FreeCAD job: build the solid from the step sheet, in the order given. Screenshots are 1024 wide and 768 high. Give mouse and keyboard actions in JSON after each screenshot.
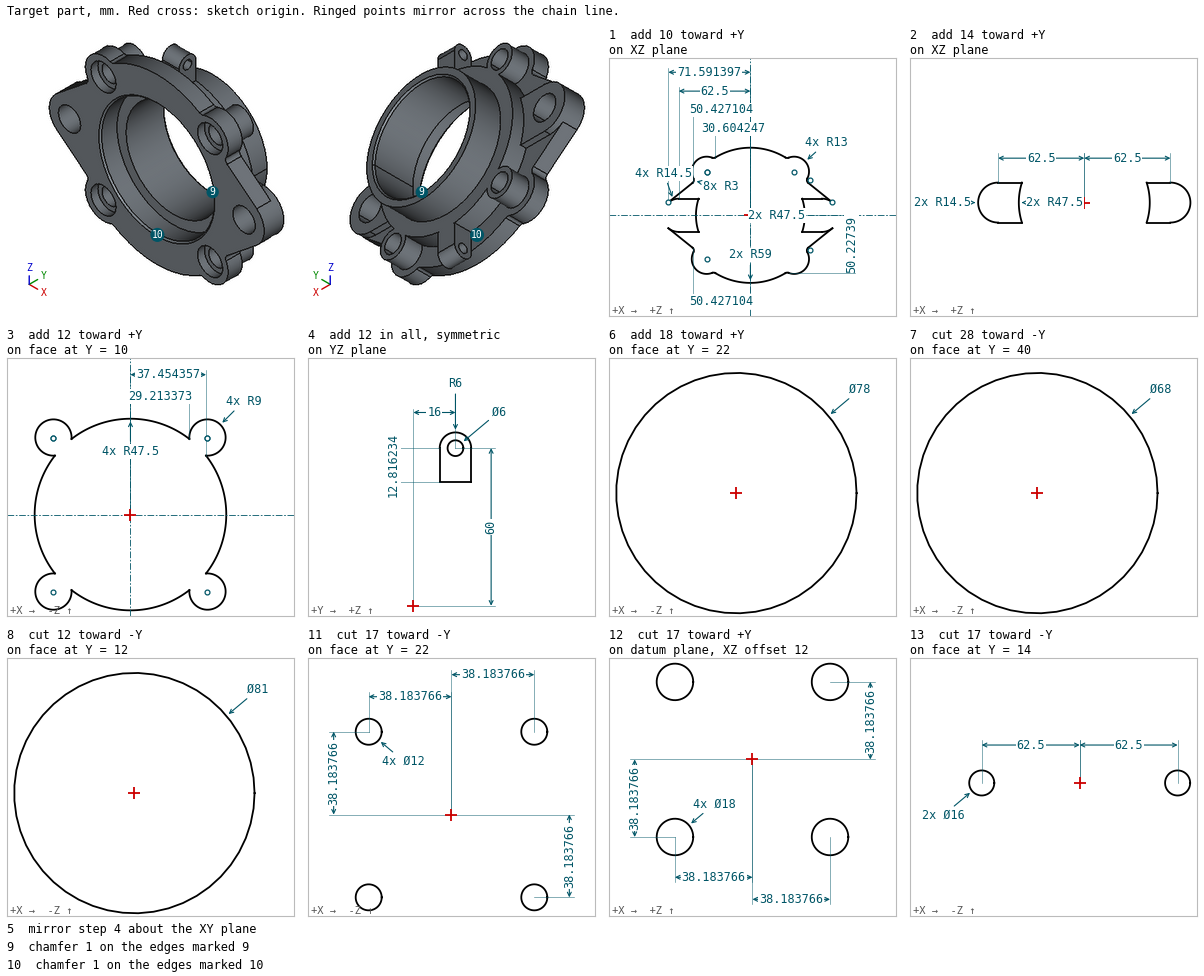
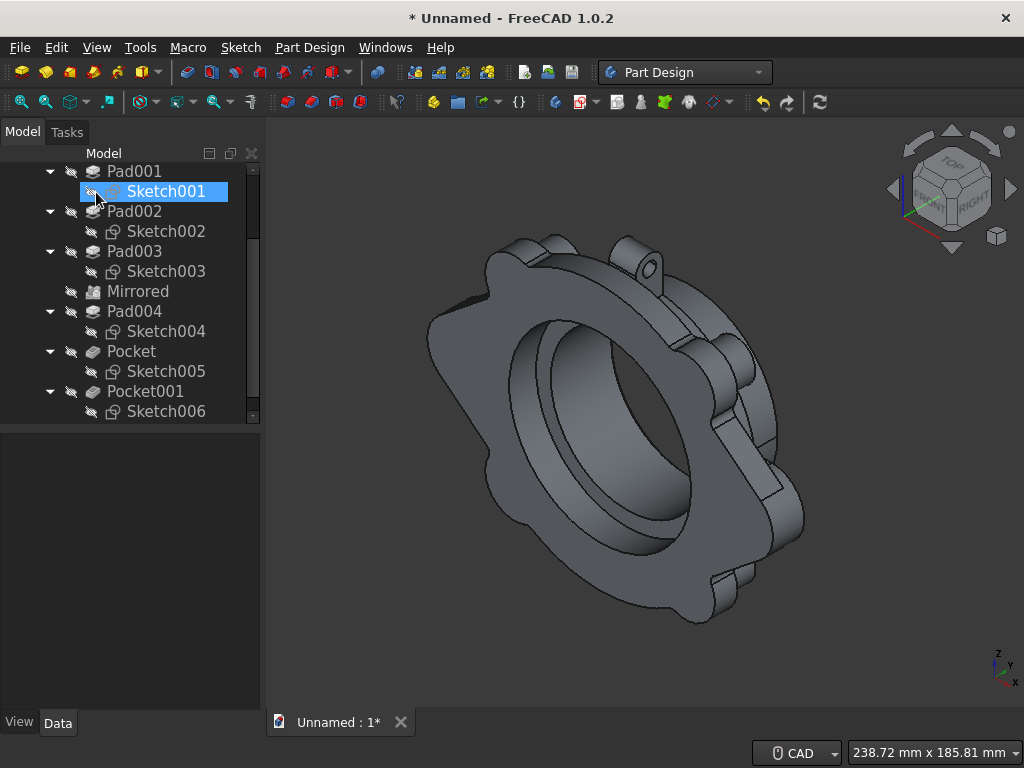
{"action": "key", "text": "v f"}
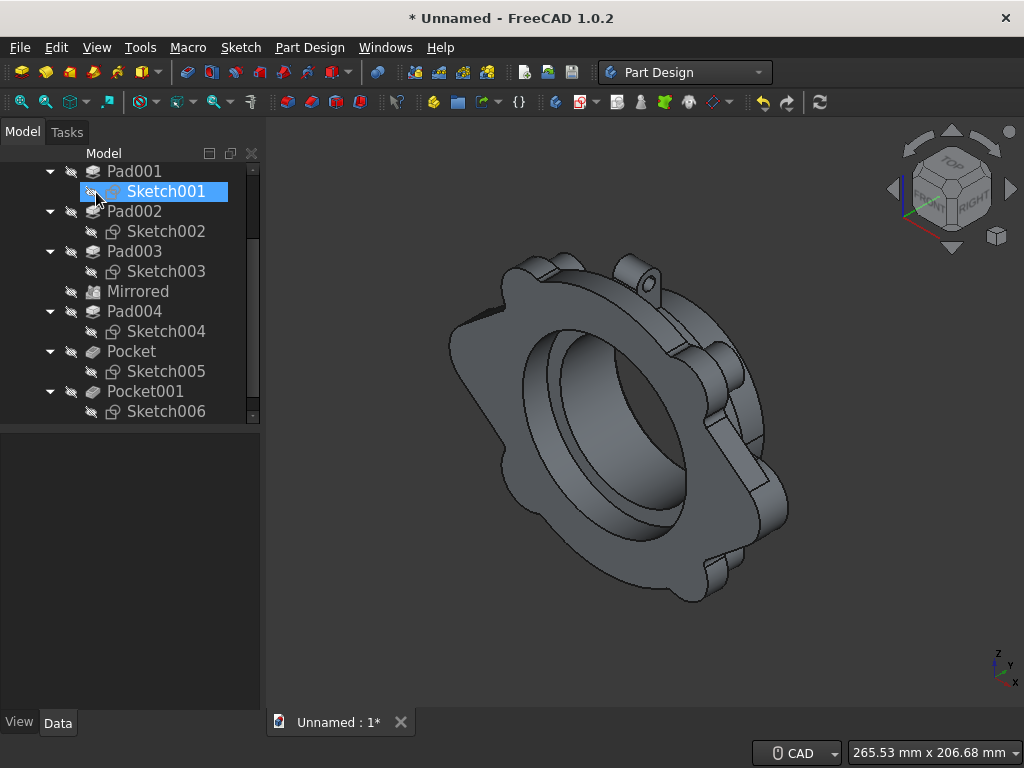
{"action": "left_click", "coordinate": [523, 387]}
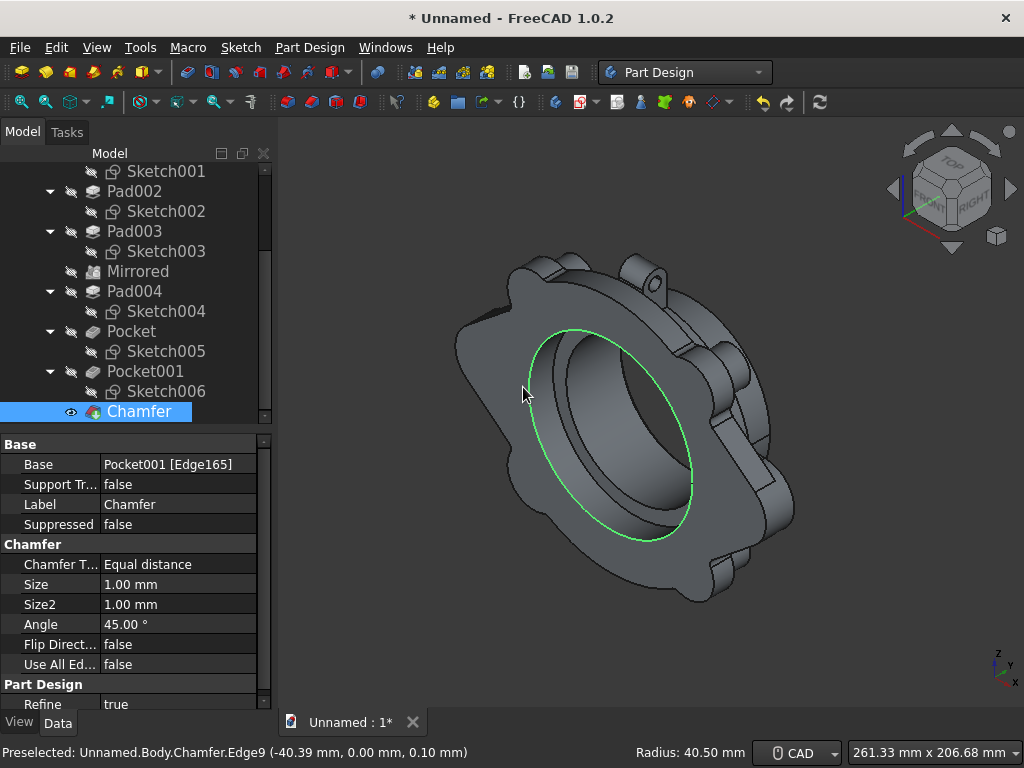
{"action": "left_click", "coordinate": [312, 102]}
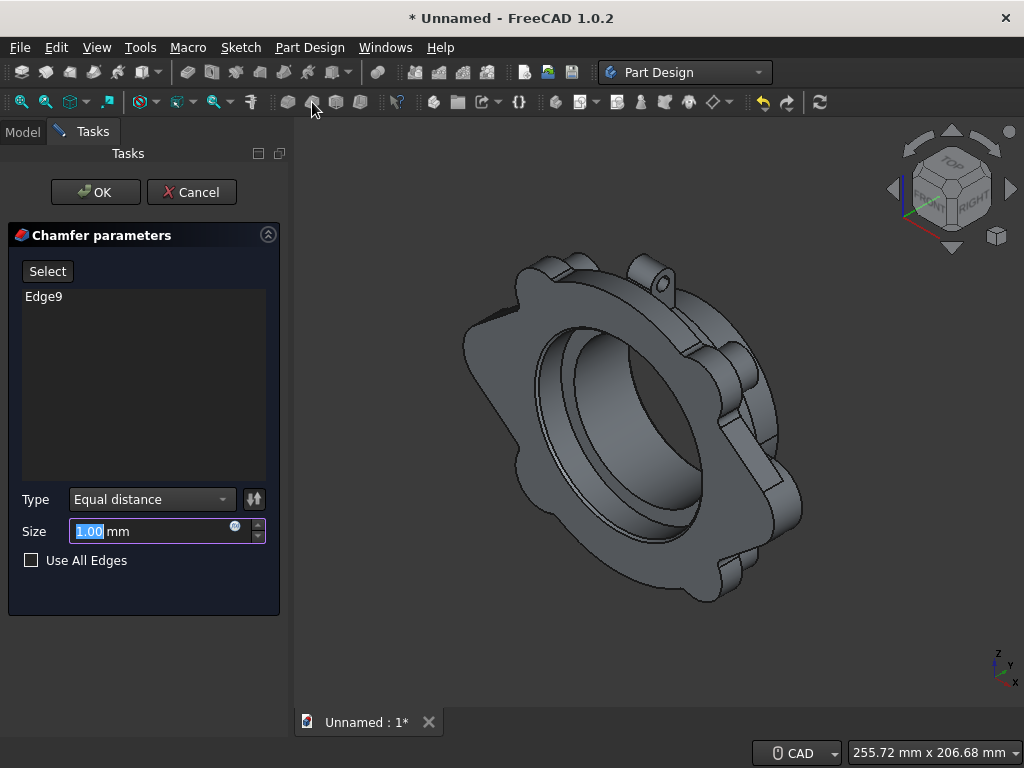
{"action": "type", "text": "1"}
{"action": "key", "text": "Tab"}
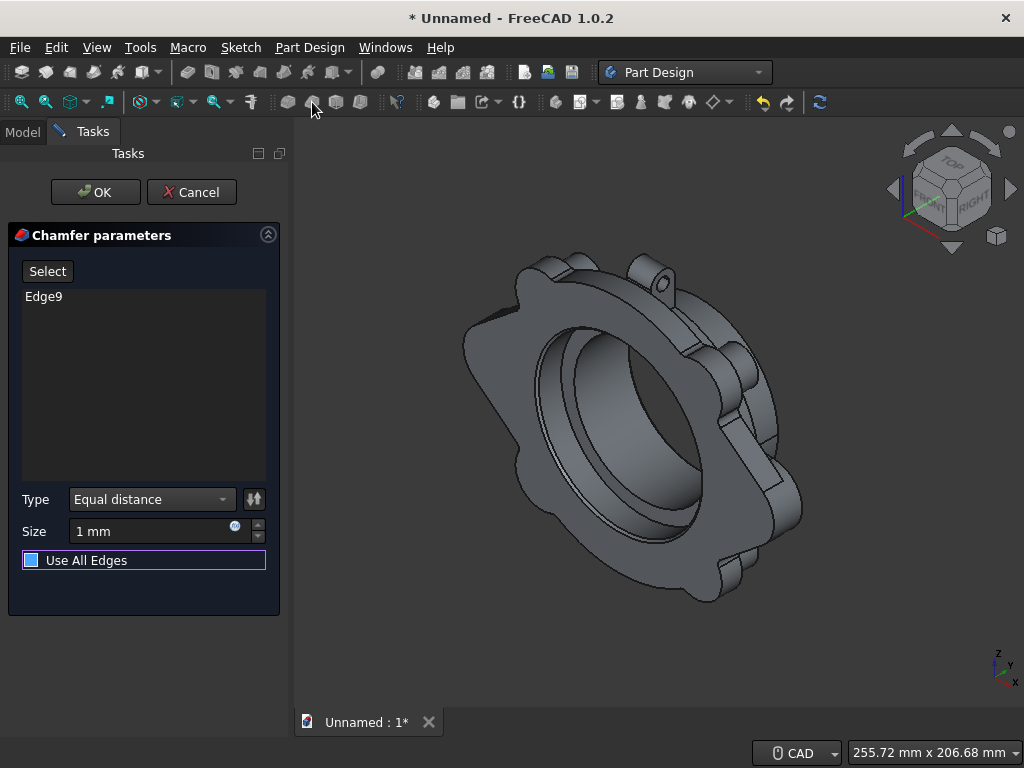
{"action": "left_click", "coordinate": [96, 192]}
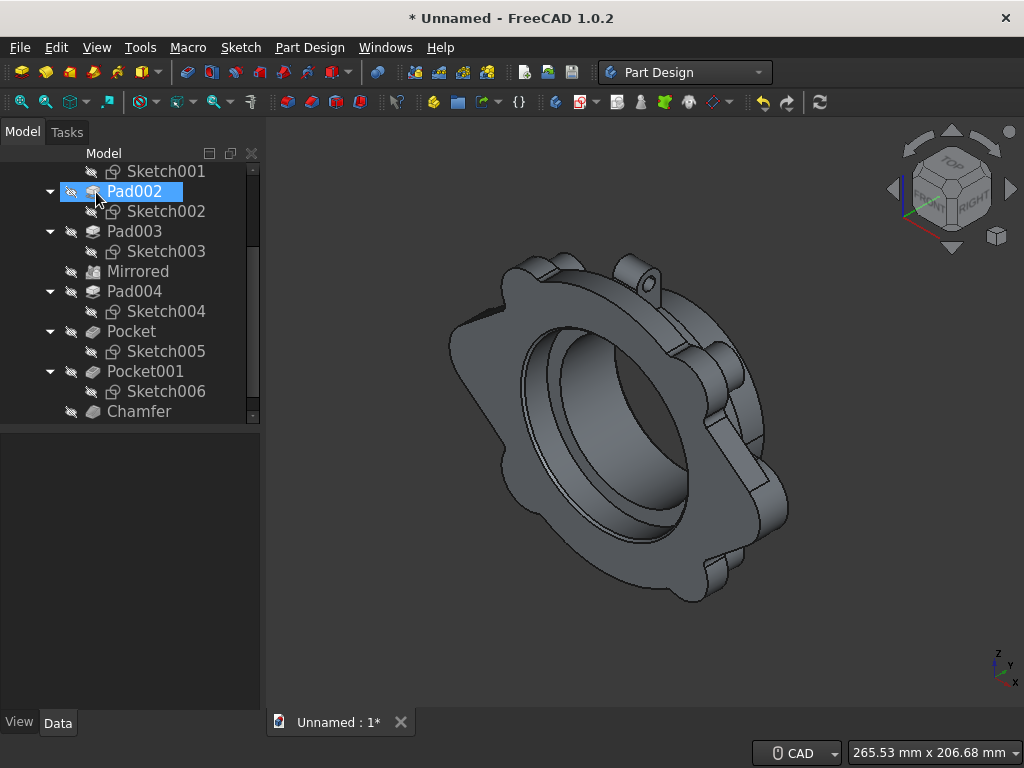
{"action": "key", "text": "4"}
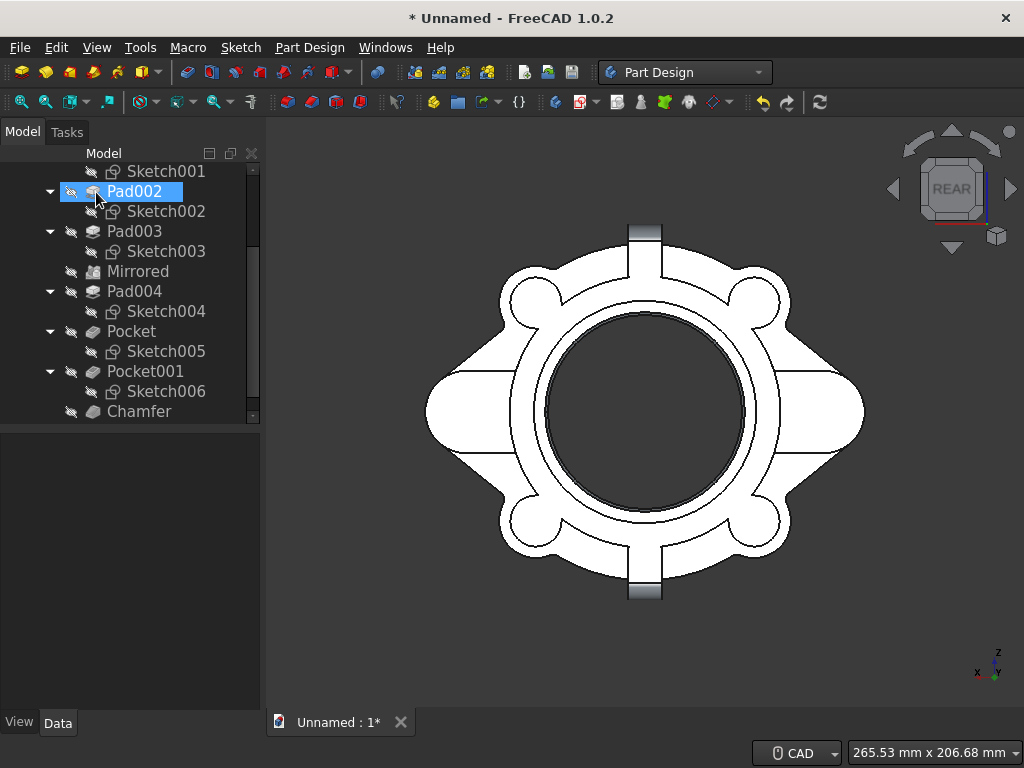
{"action": "left_click", "coordinate": [645, 558]}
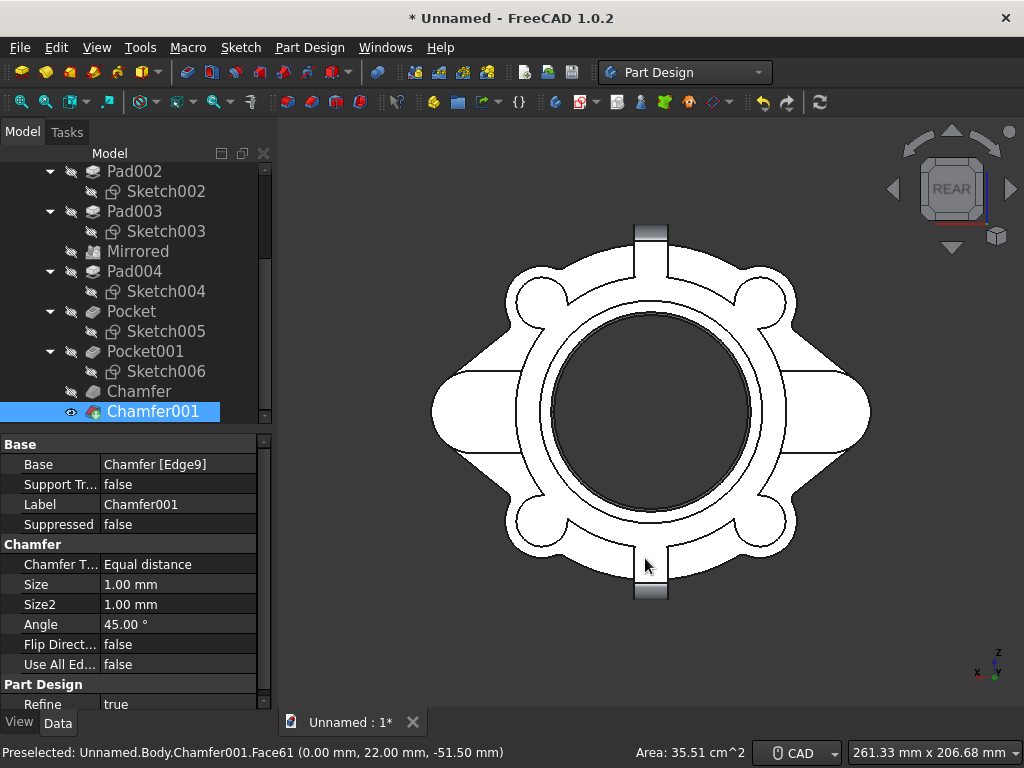
{"action": "left_click", "coordinate": [580, 102]}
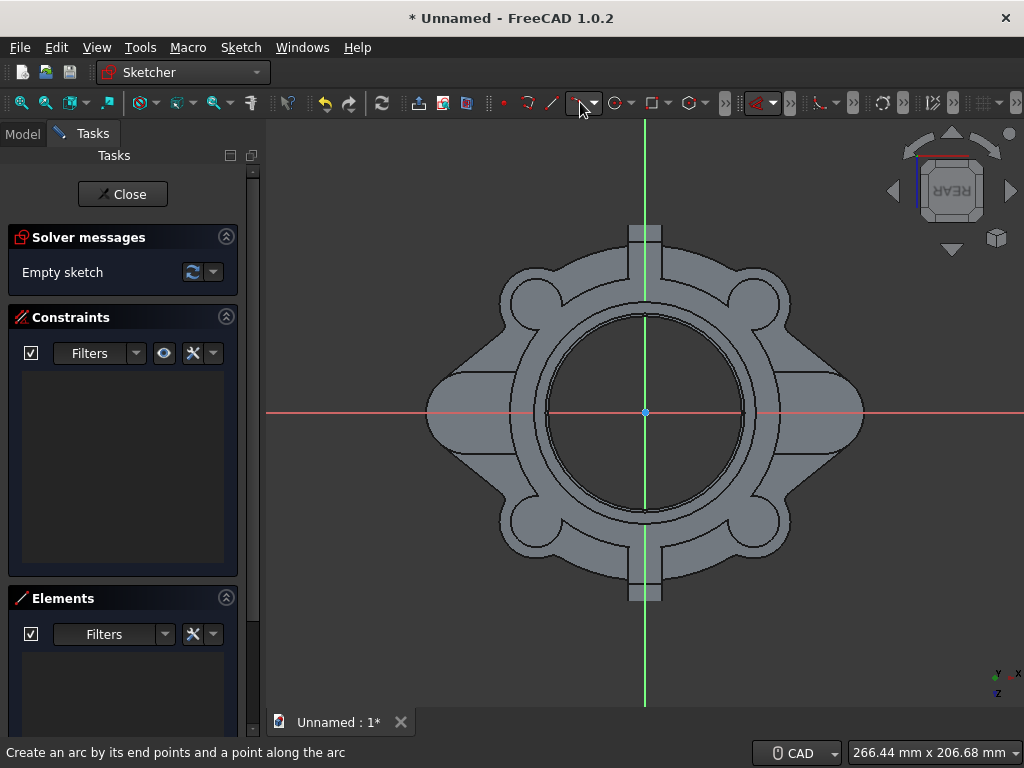
{"action": "scroll", "coordinate": [784, 413], "scroll_direction": "up", "scroll_amount": 2}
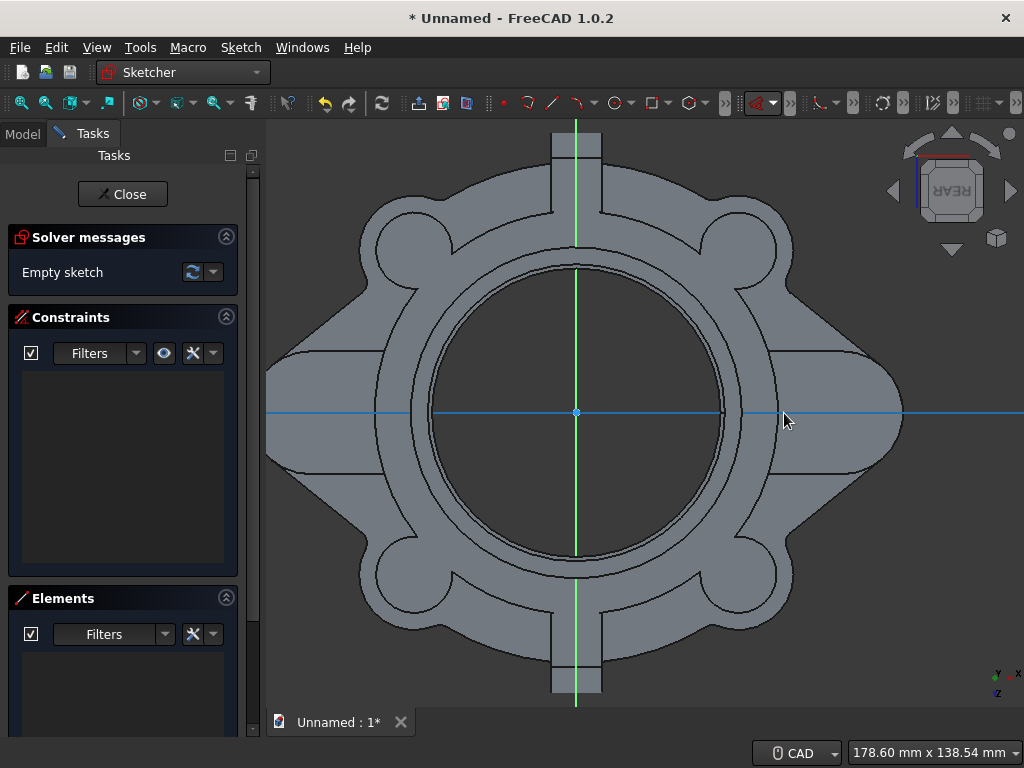
{"action": "key", "text": "g c"}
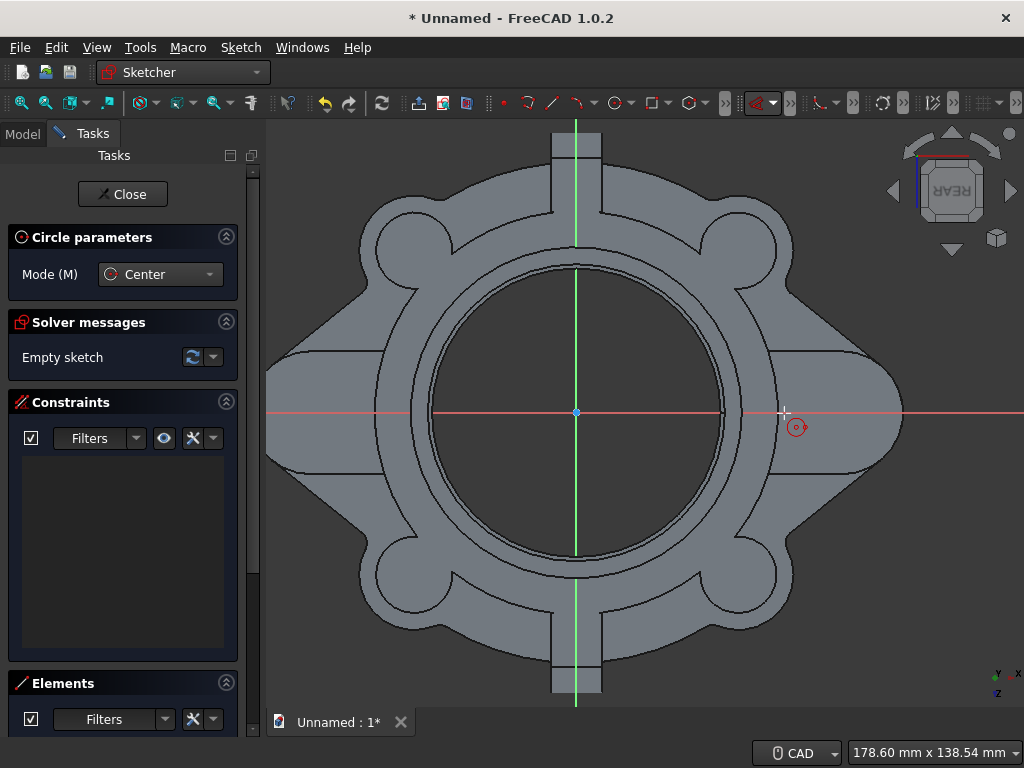
{"action": "left_click", "coordinate": [414, 251]}
{"action": "left_click", "coordinate": [432, 233]}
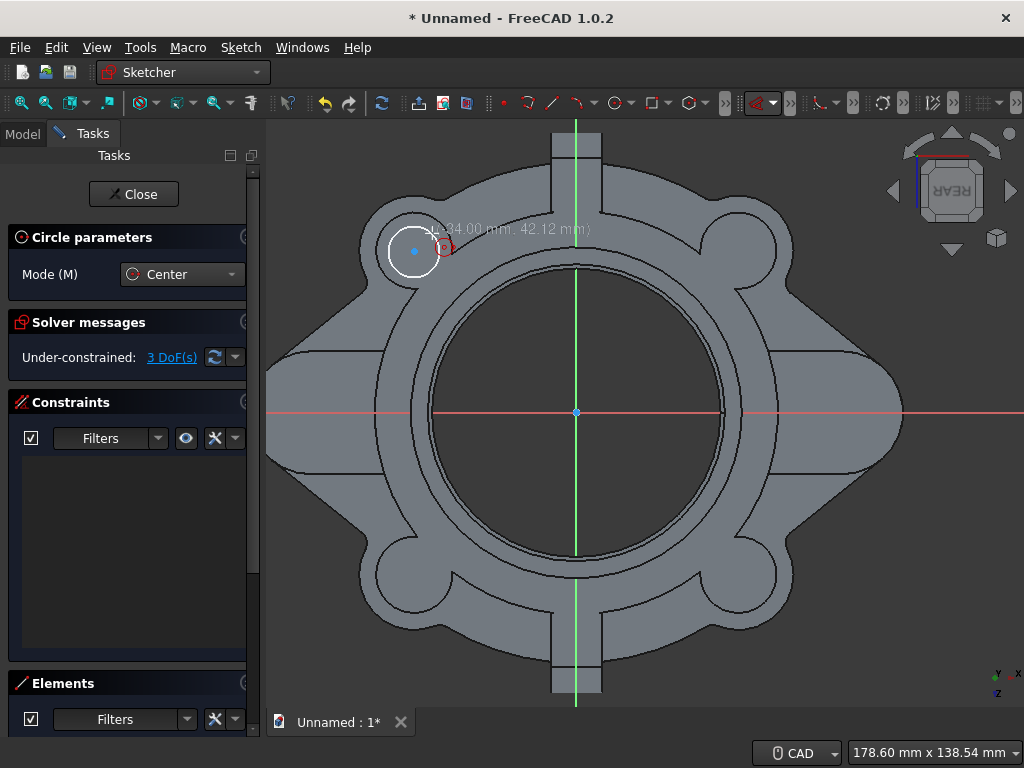
{"action": "left_click", "coordinate": [738, 251]}
{"action": "left_click", "coordinate": [756, 233]}